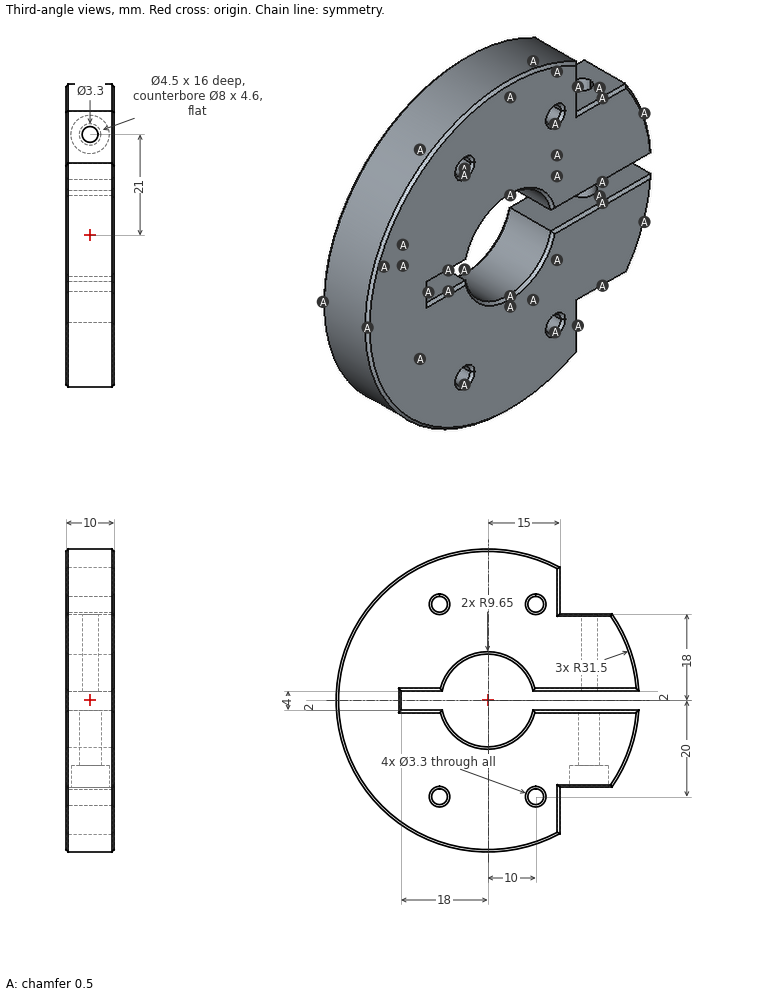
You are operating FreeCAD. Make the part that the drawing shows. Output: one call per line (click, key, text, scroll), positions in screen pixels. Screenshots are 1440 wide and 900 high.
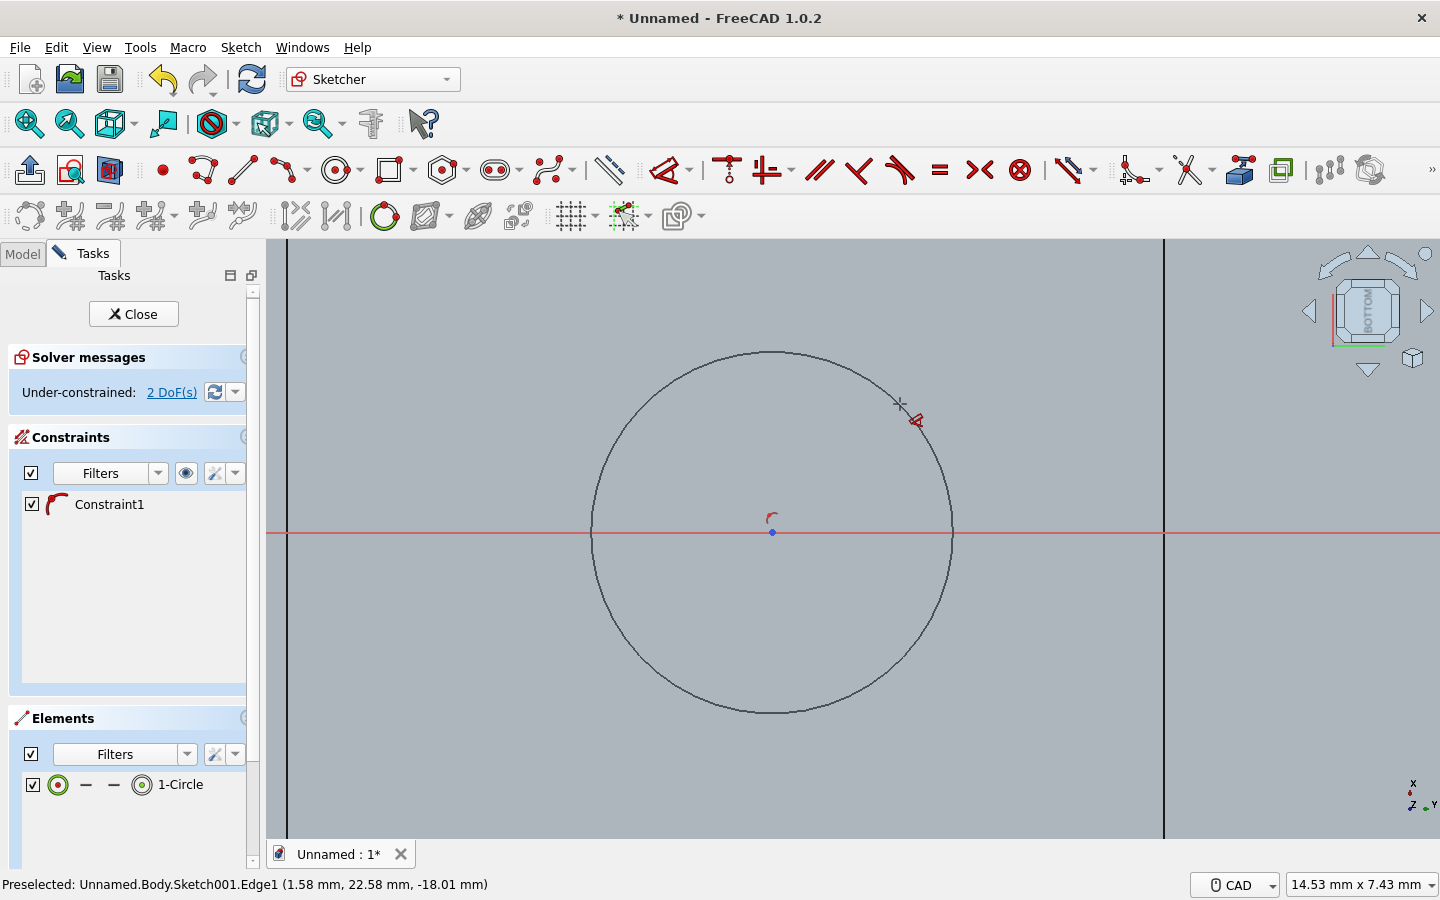
click(899, 404)
click(921, 381)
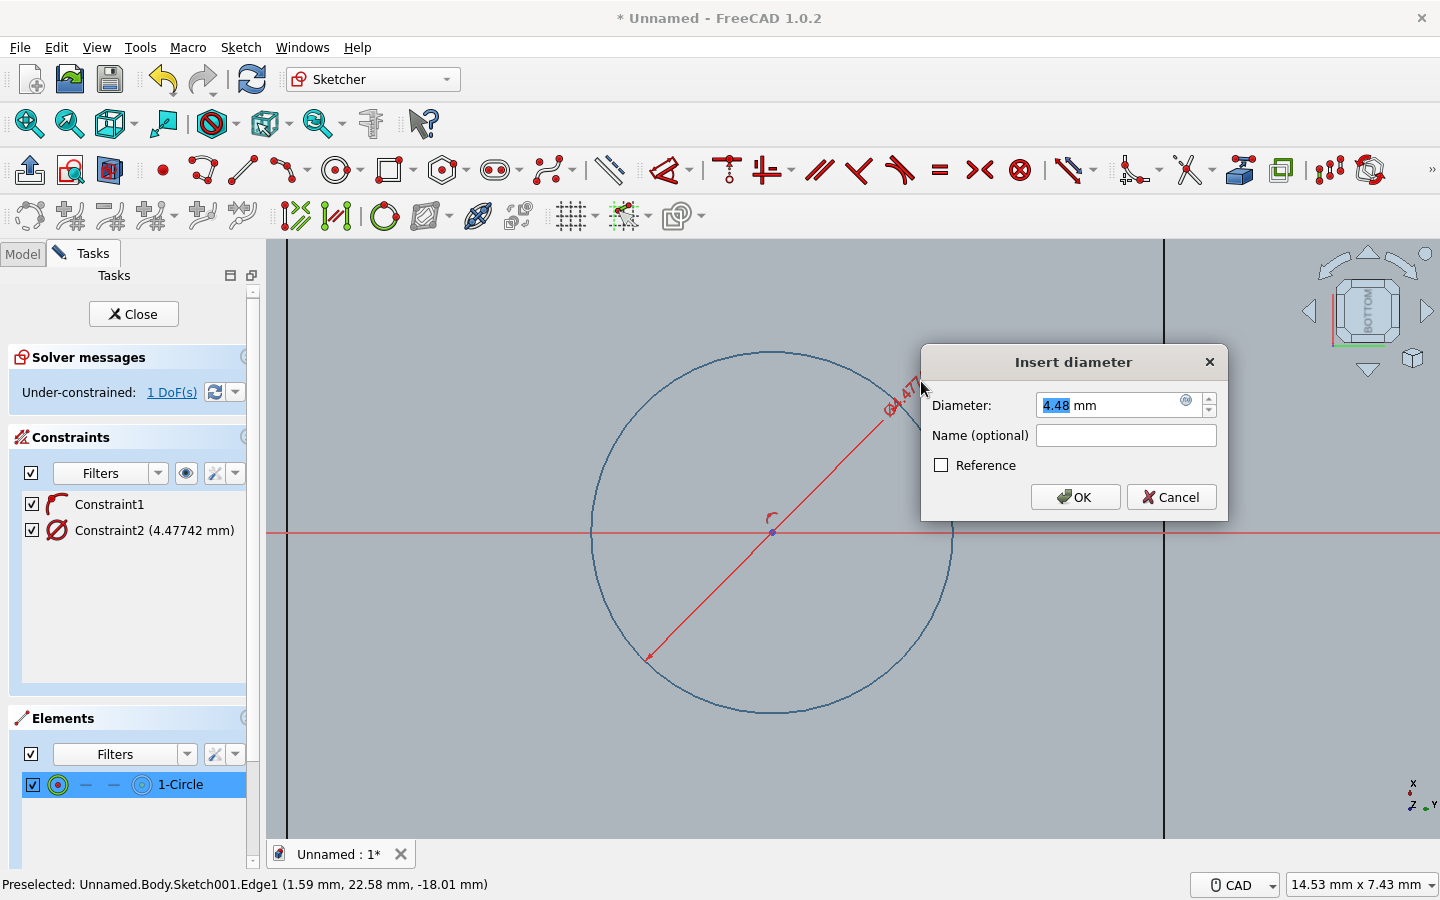
text(4.5)
key(Return)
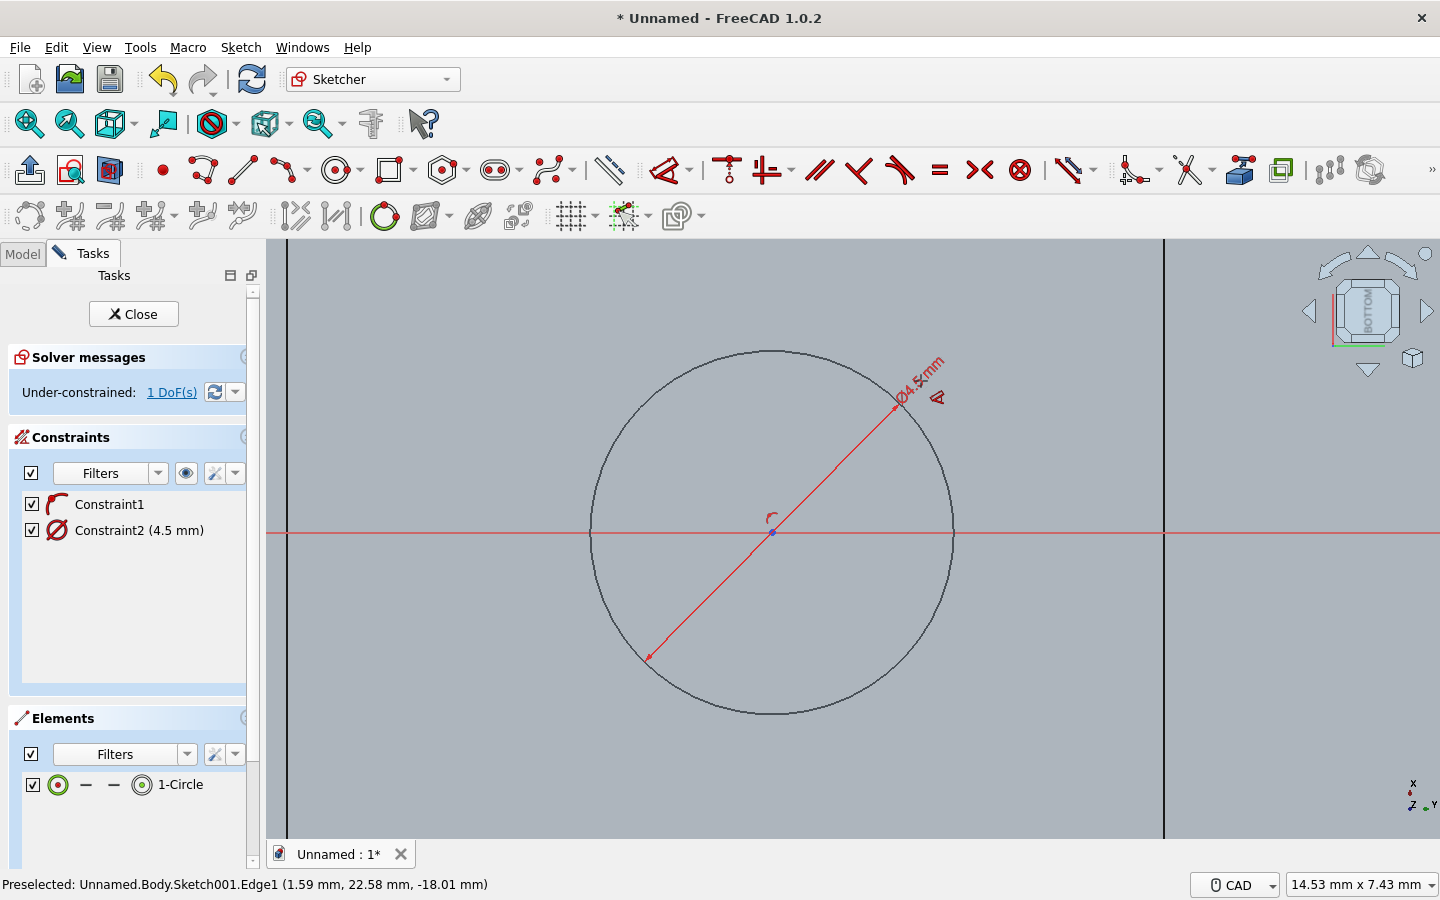
click(772, 533)
click(533, 567)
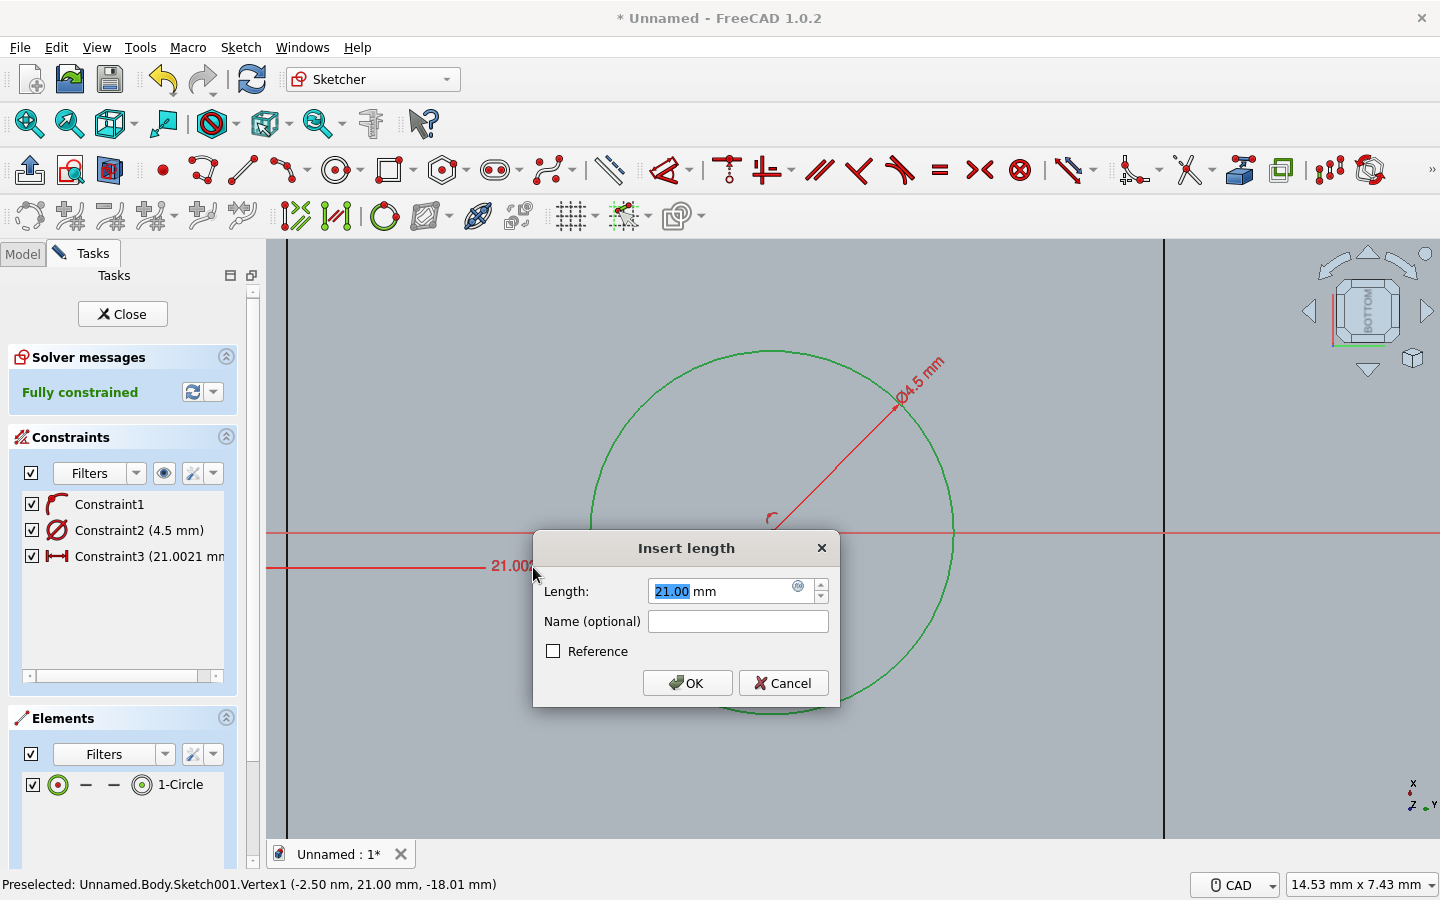
text(21)
key(Return)
key(Escape)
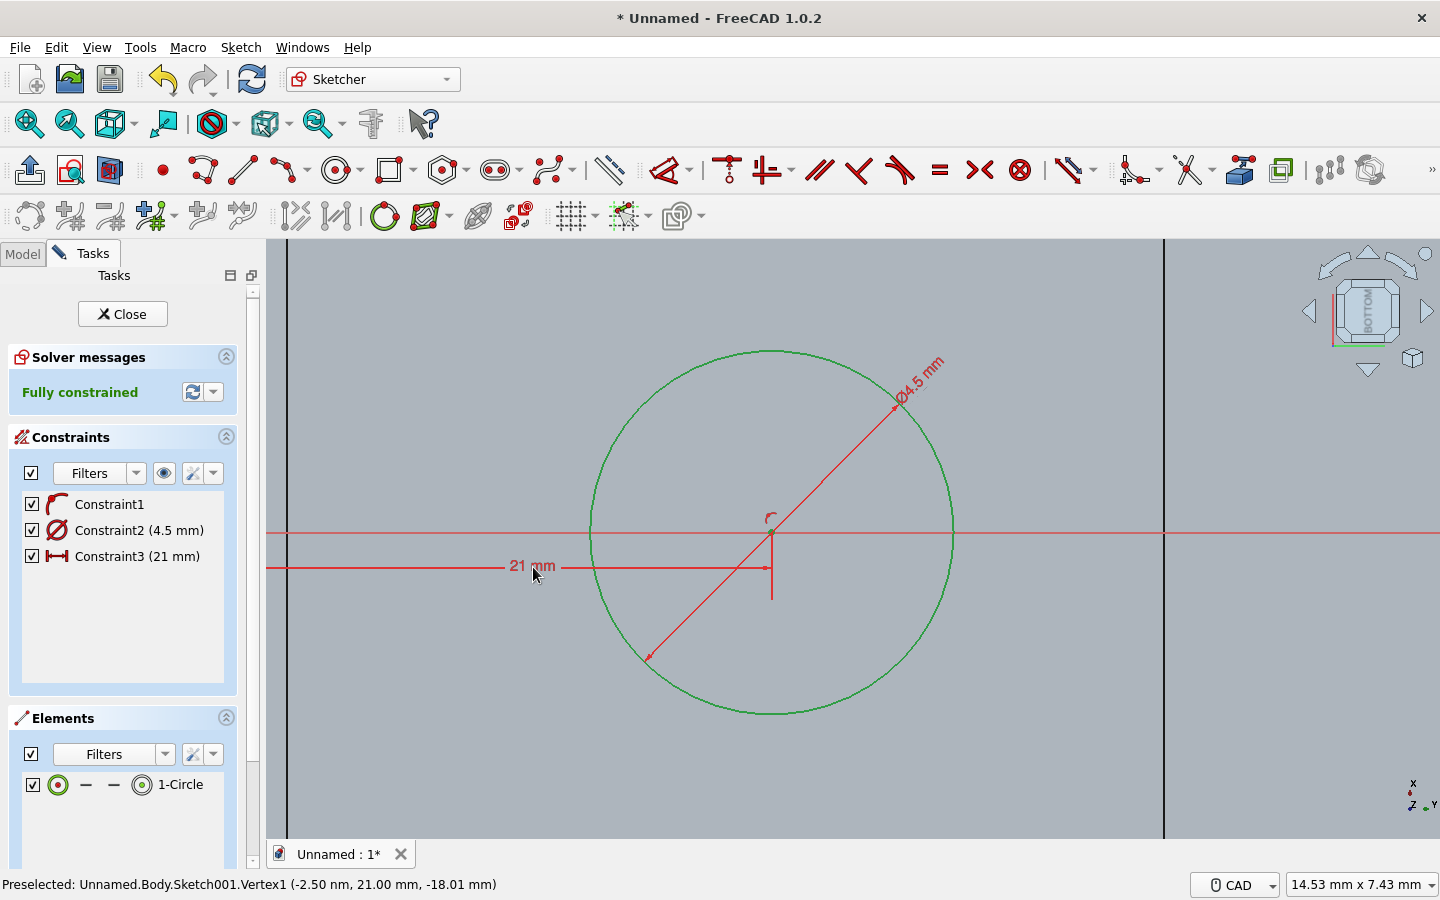
click(123, 314)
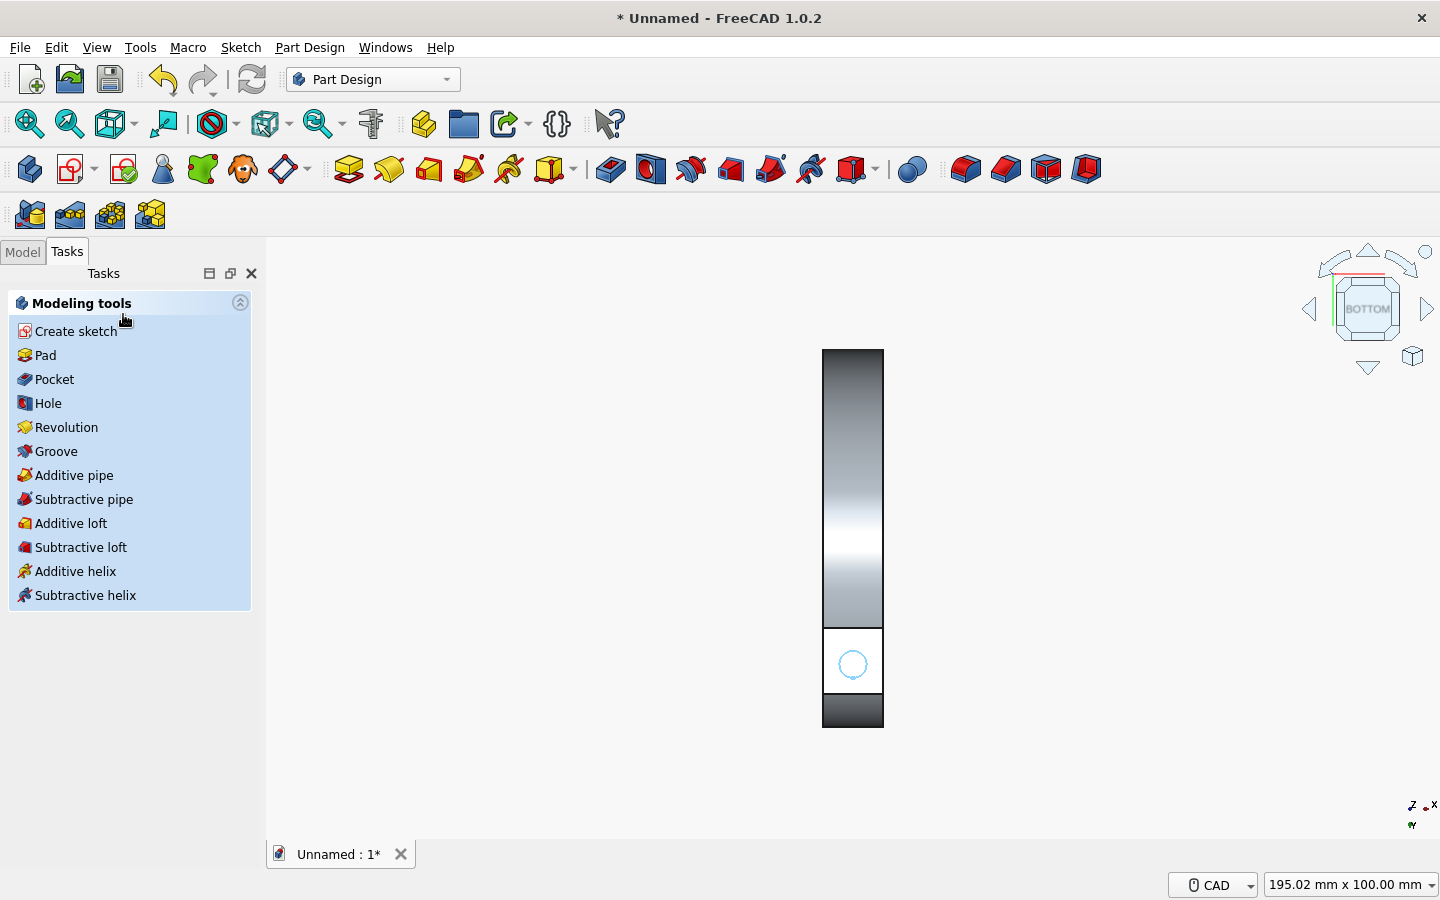
click(652, 170)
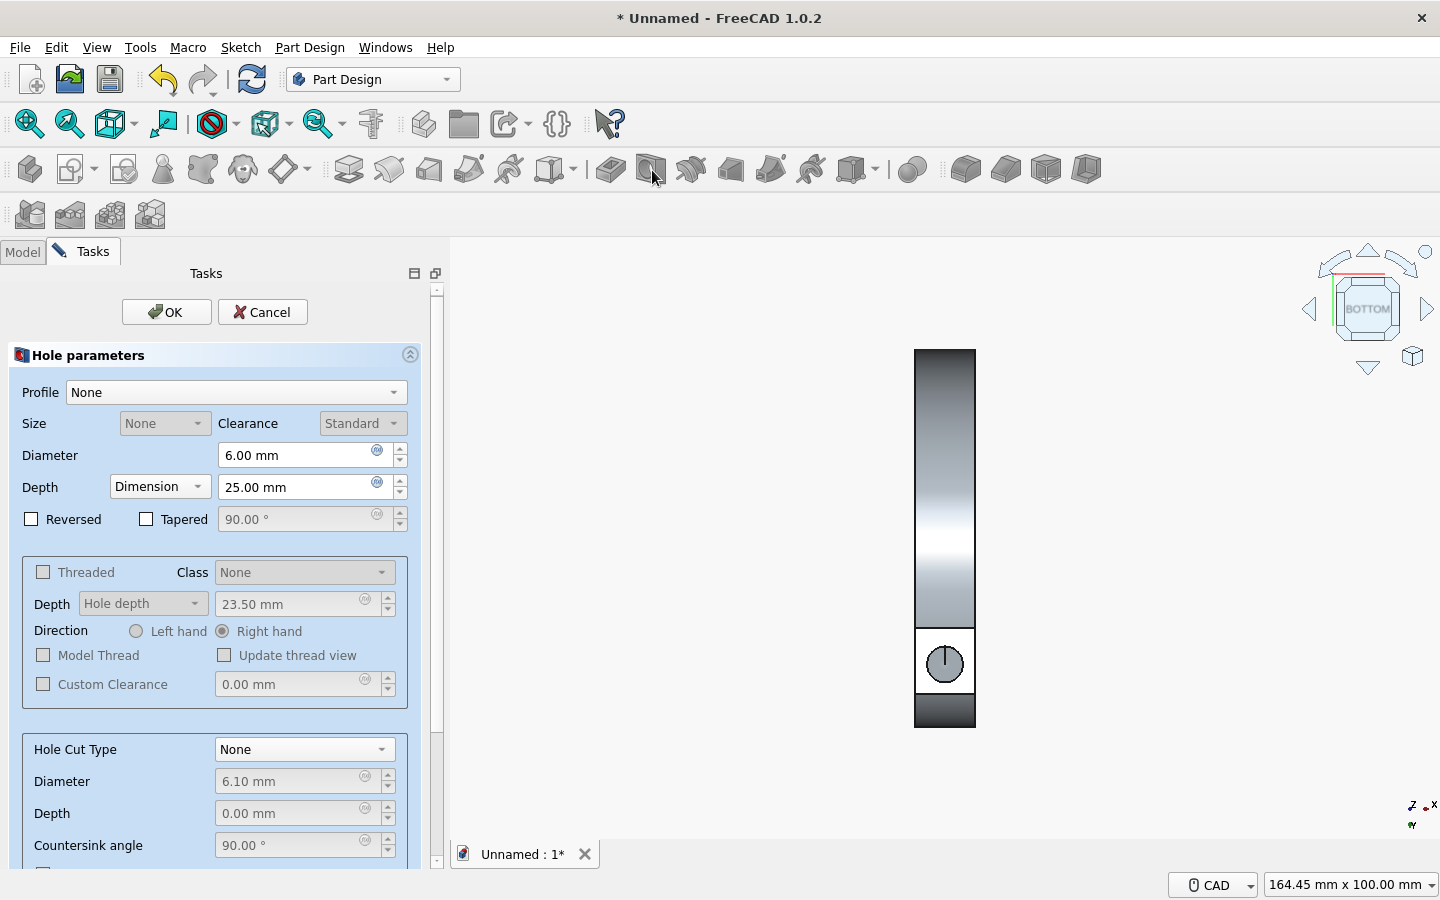
triple_click(305, 455)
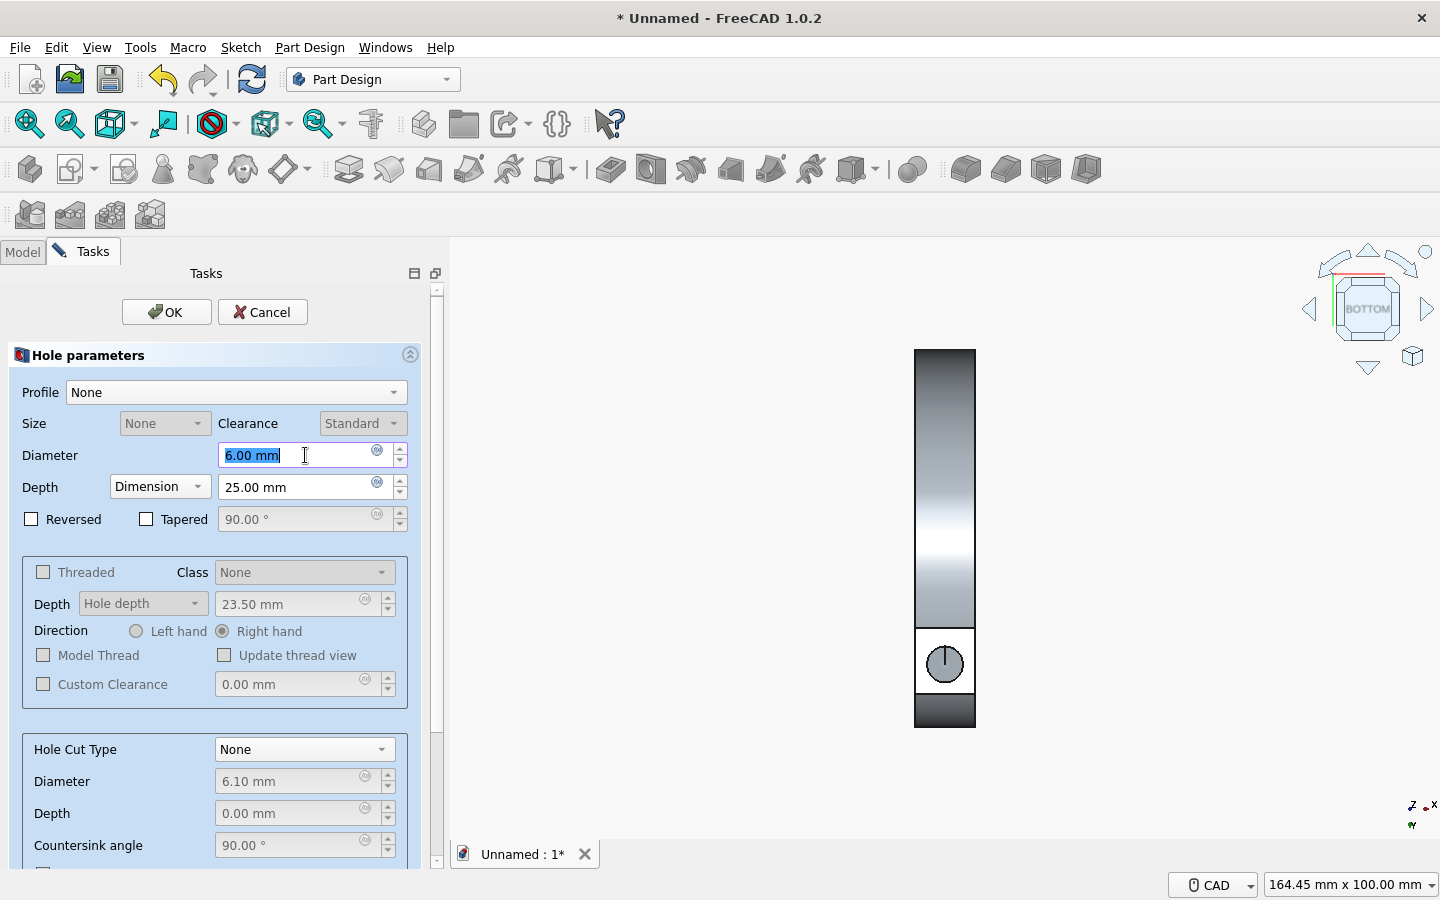
text(4.5)
key(Tab)